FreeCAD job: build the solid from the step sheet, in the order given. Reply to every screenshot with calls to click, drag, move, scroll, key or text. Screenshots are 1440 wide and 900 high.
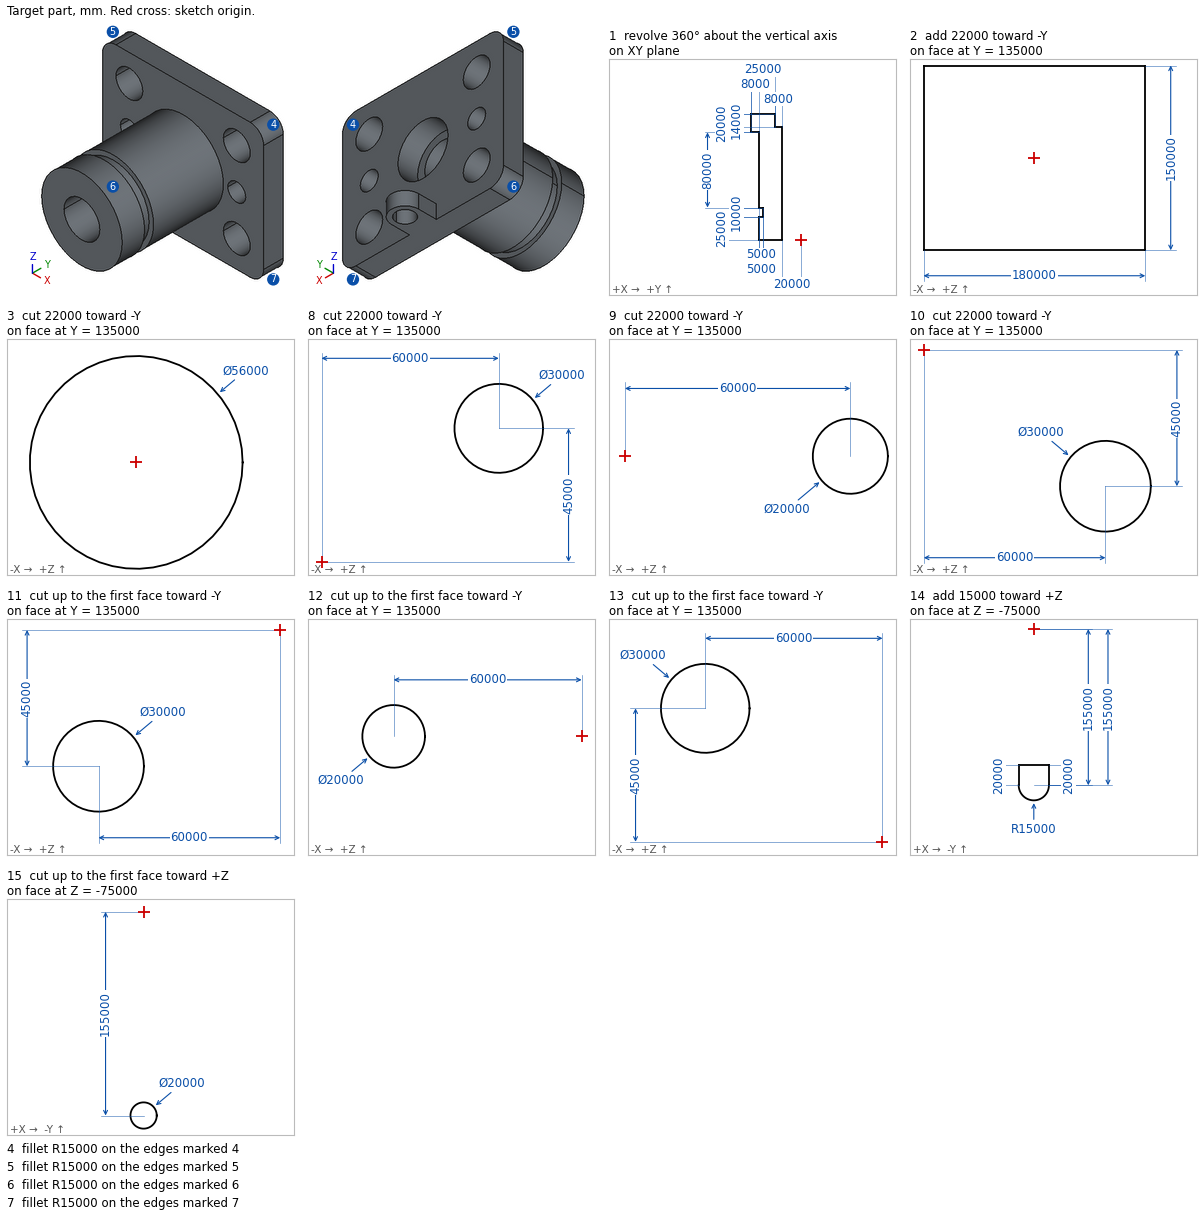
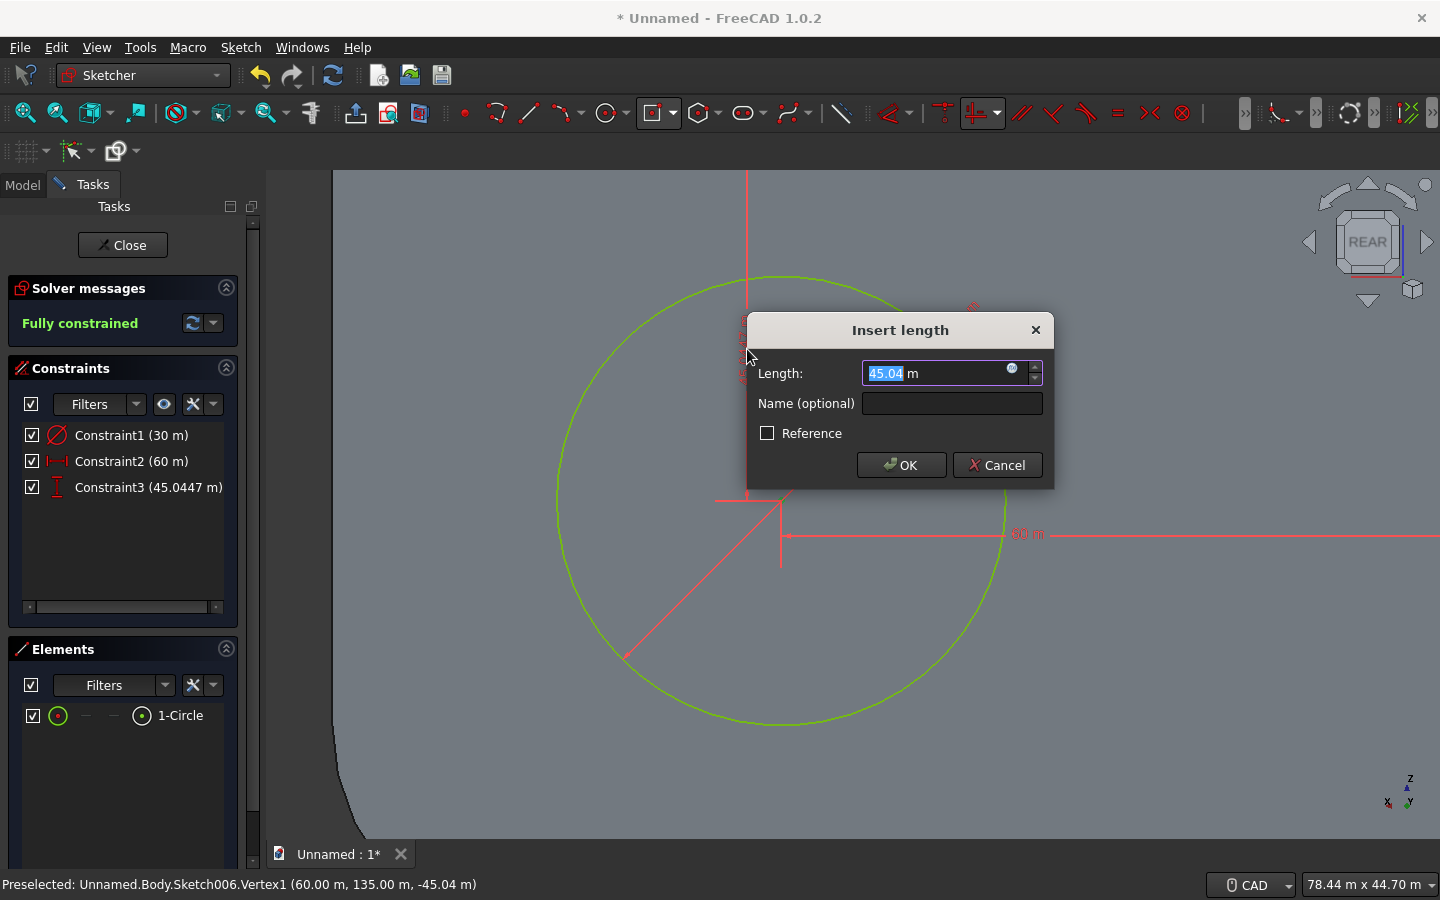
key(ctrl+a)
text(45000 mm)
key(Return)
key(Escape)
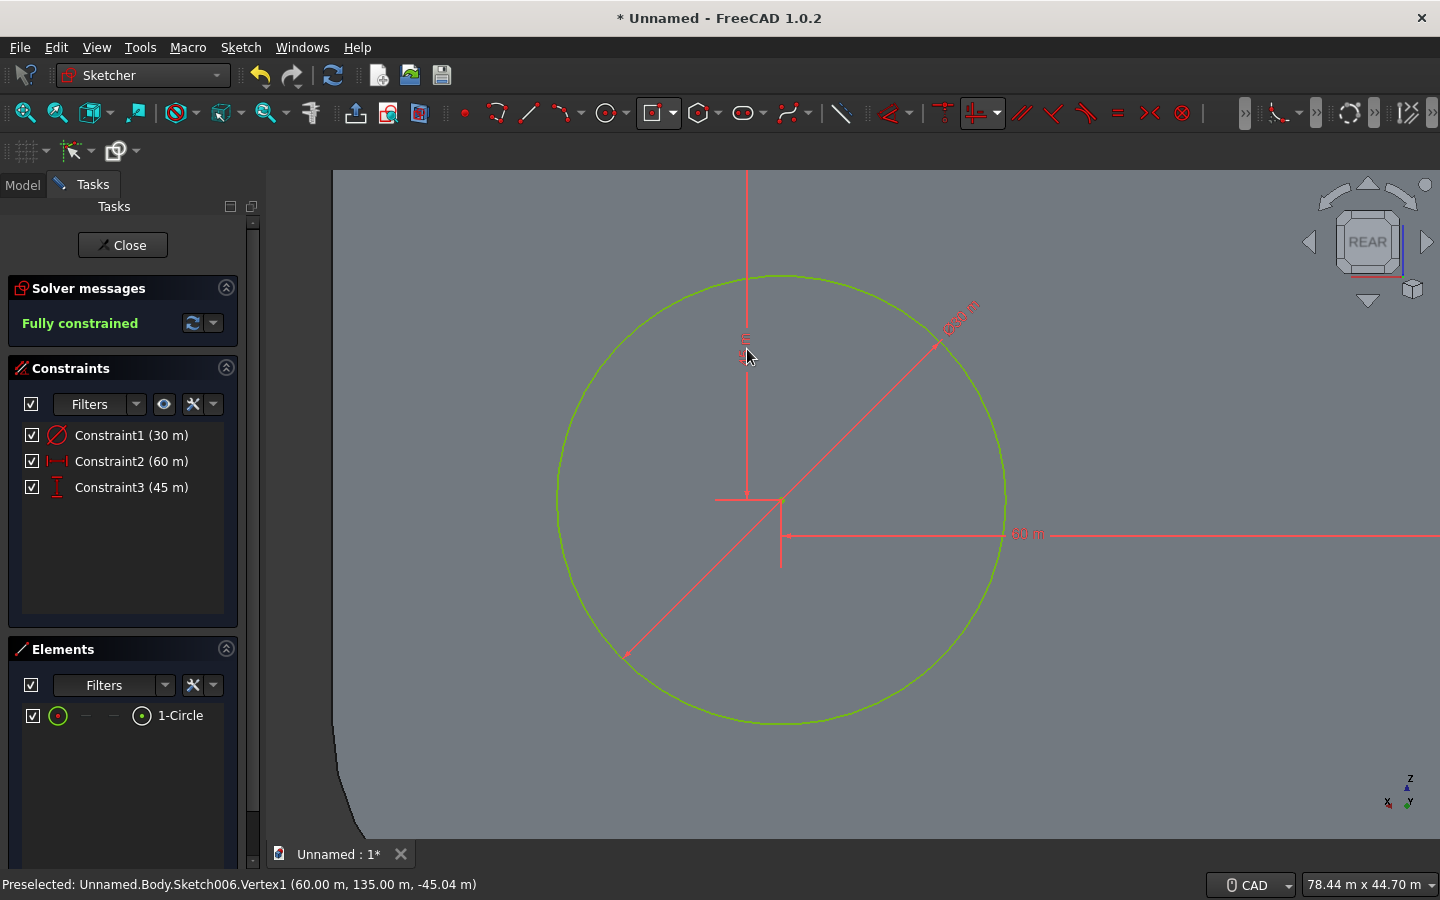
click(123, 245)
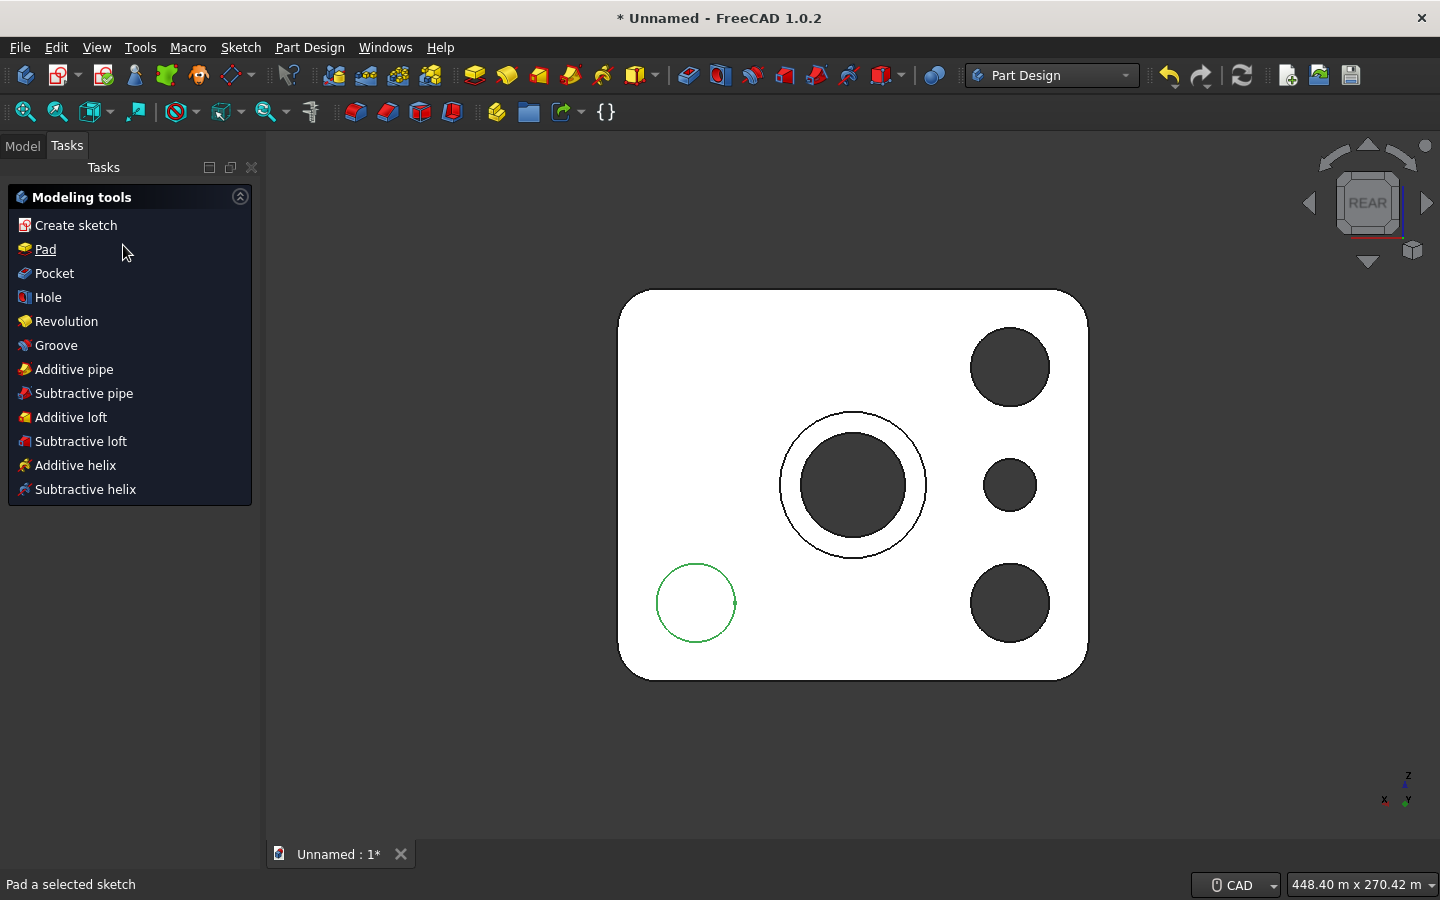
click(690, 76)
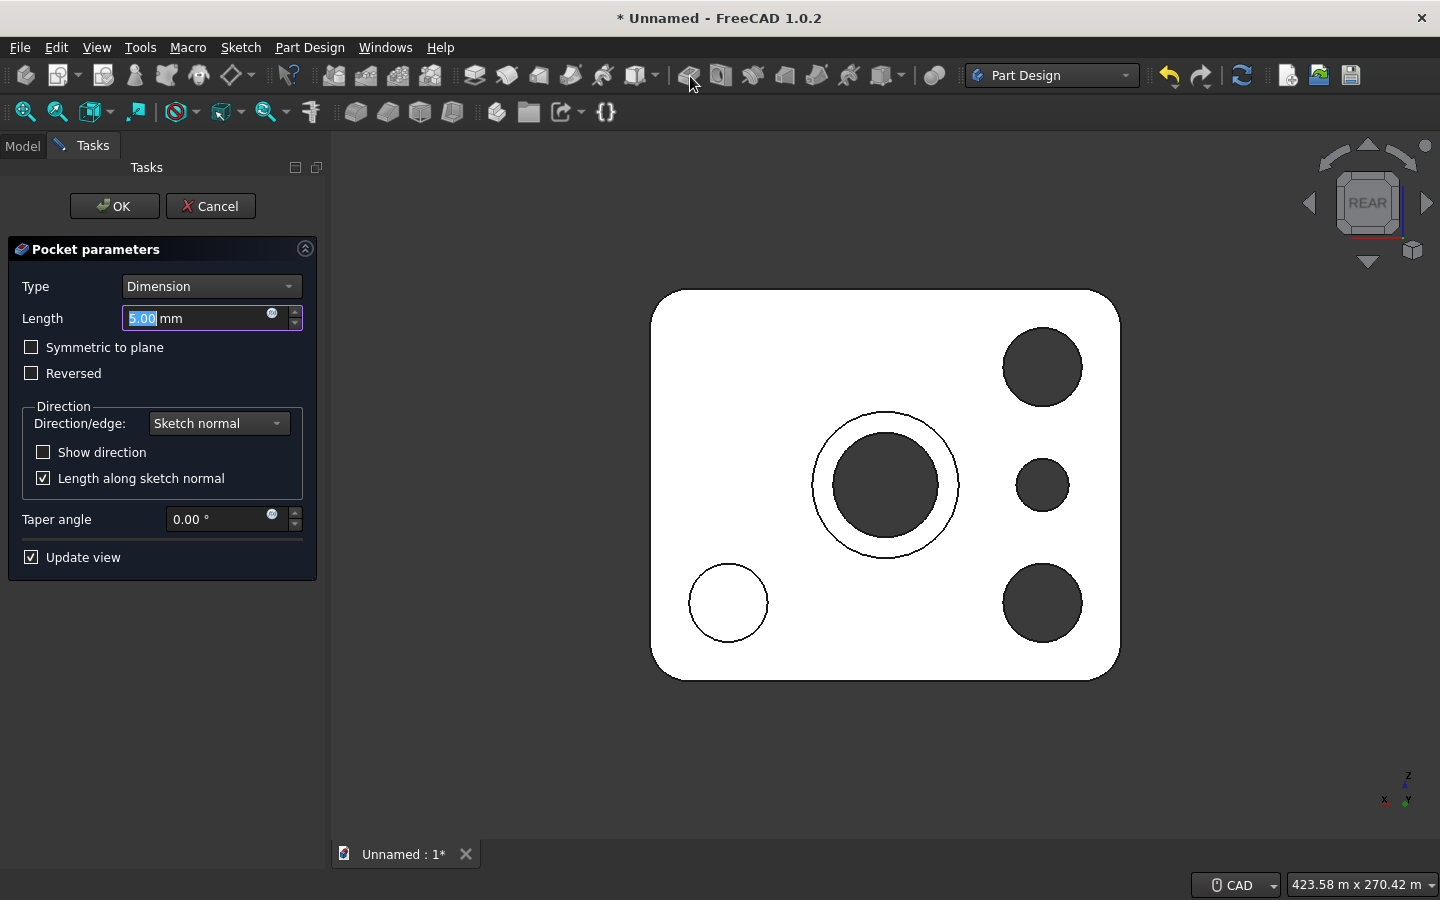
click(212, 286)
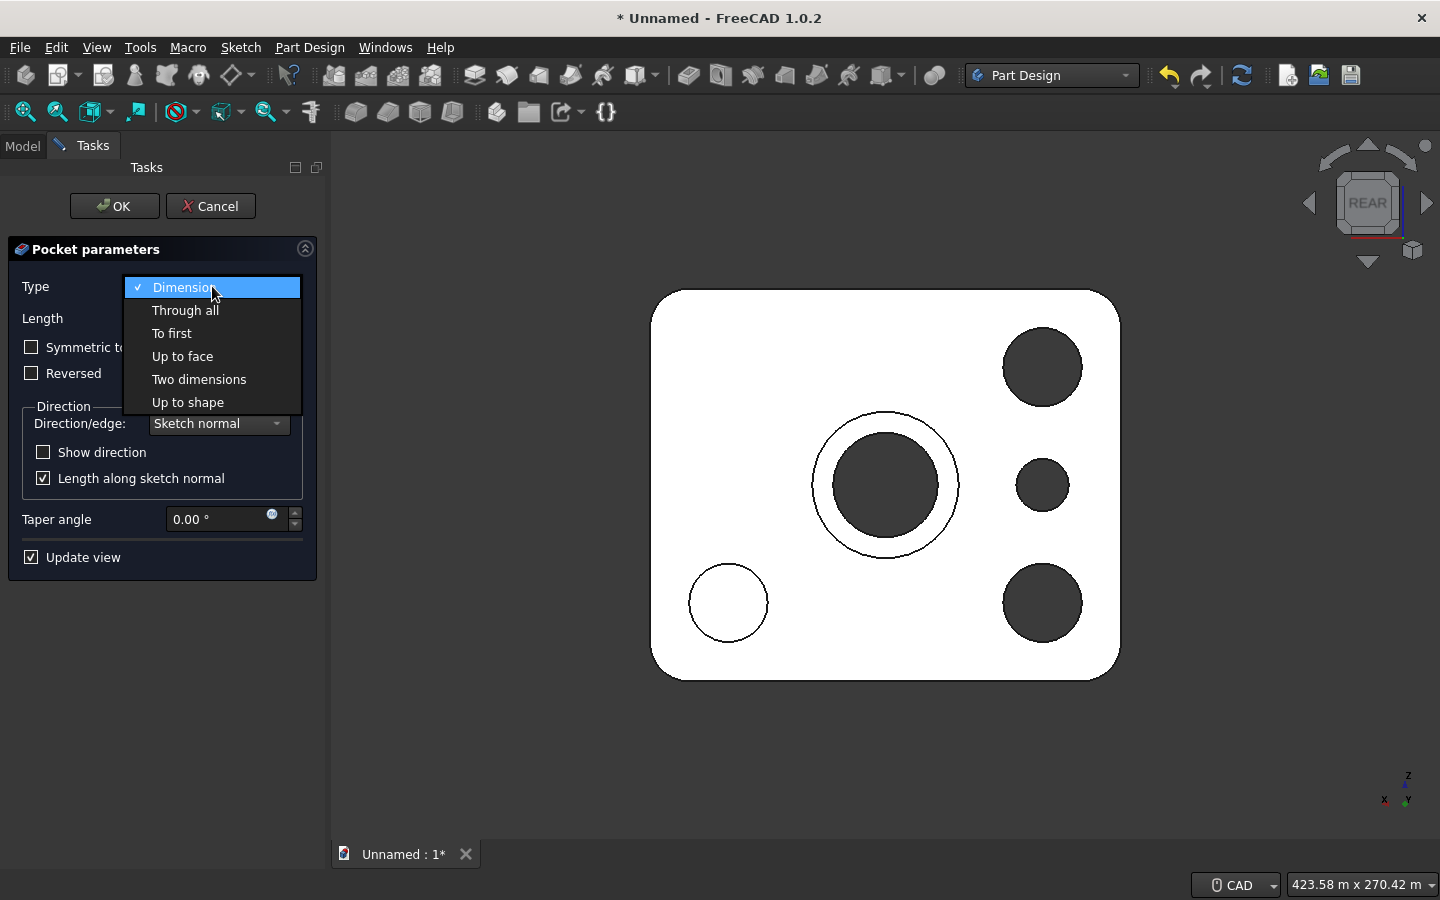
click(212, 334)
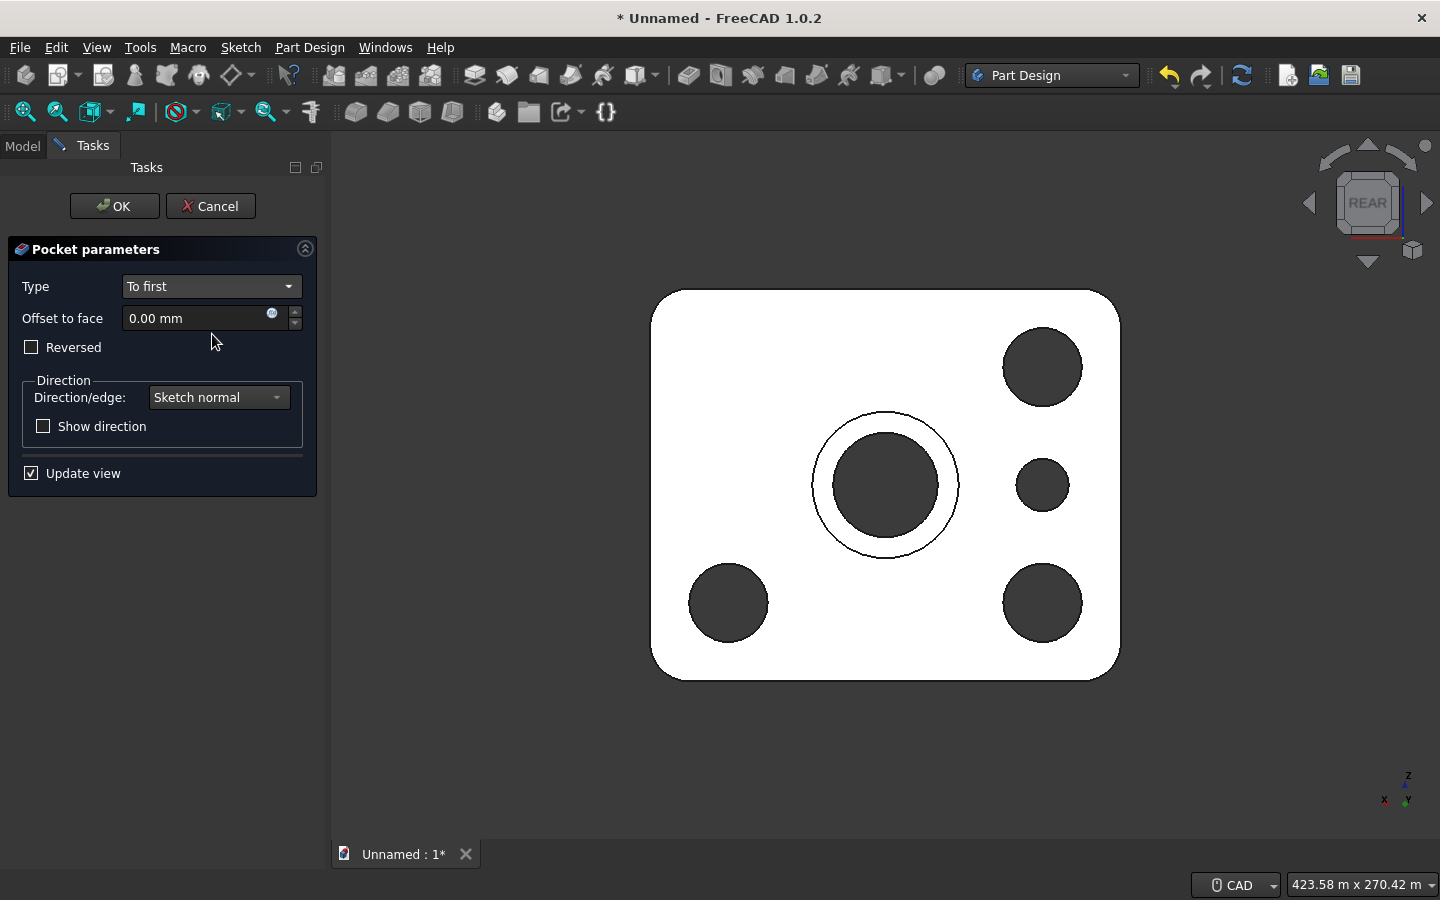
click(115, 206)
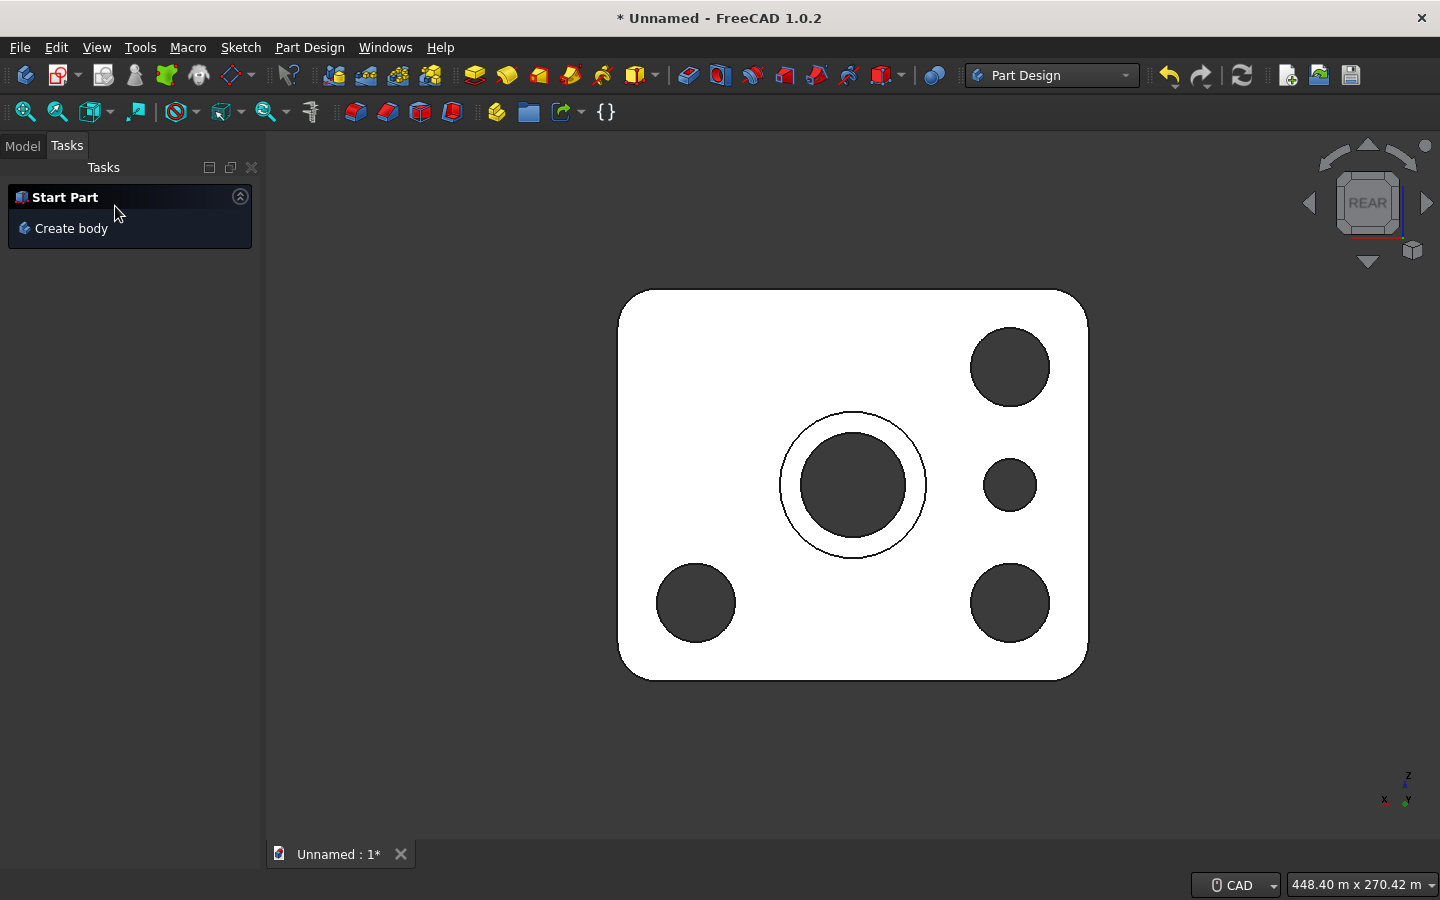
click(718, 372)